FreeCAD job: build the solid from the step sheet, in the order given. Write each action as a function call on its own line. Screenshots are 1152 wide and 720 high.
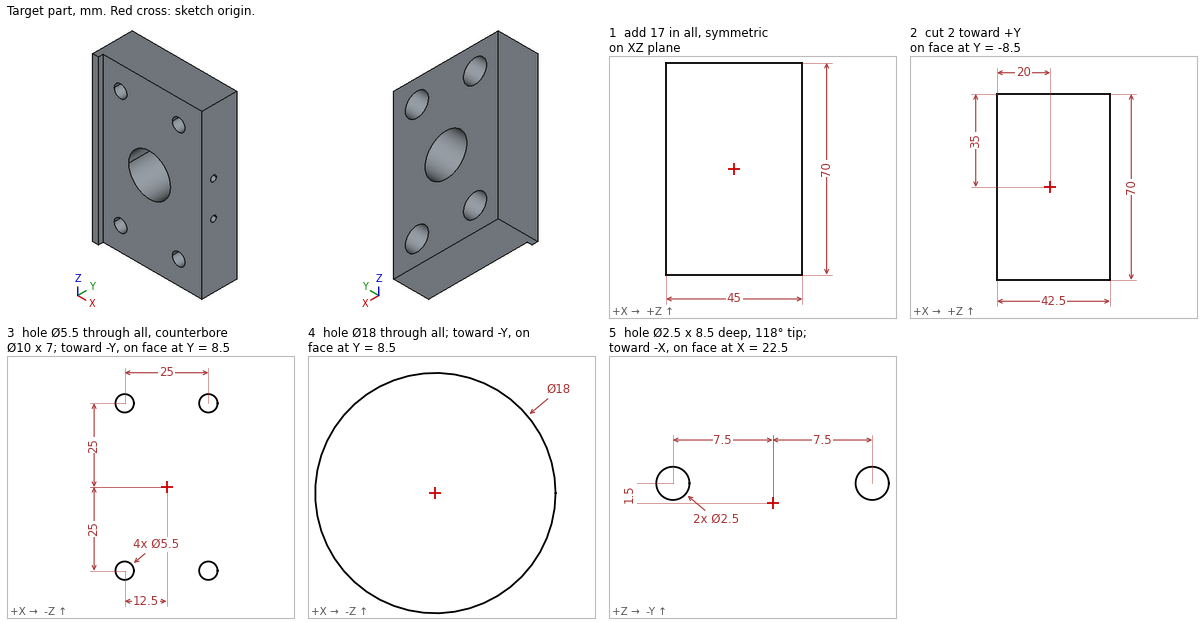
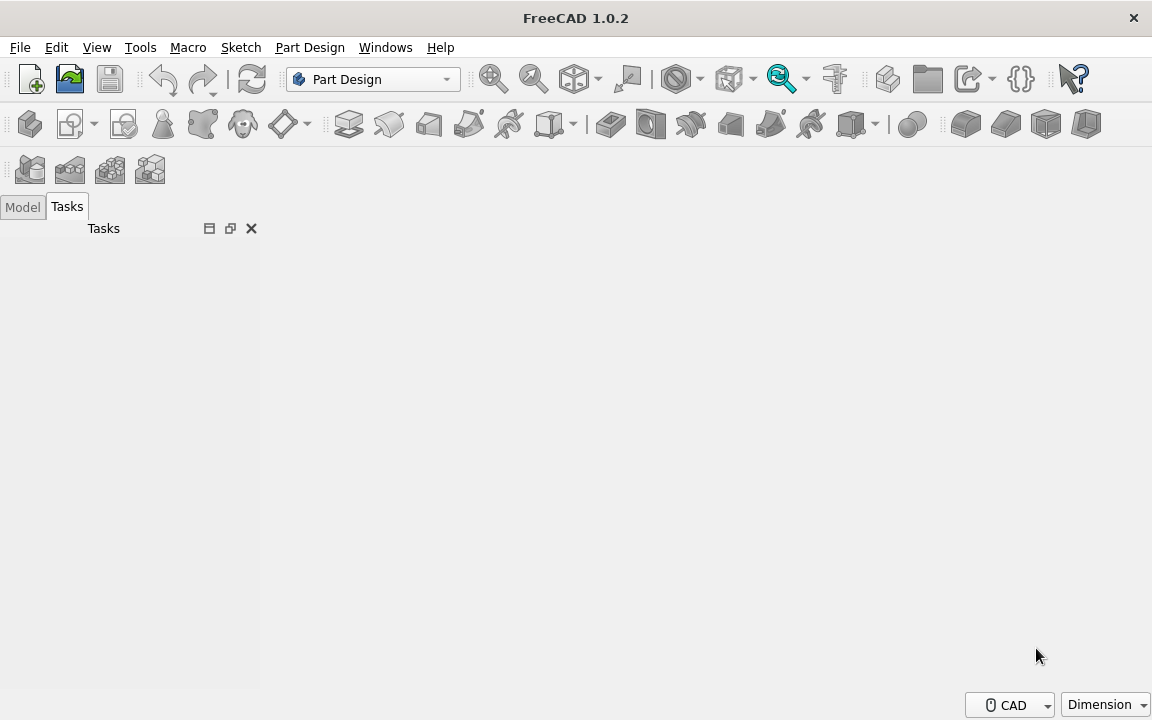
click(30, 80)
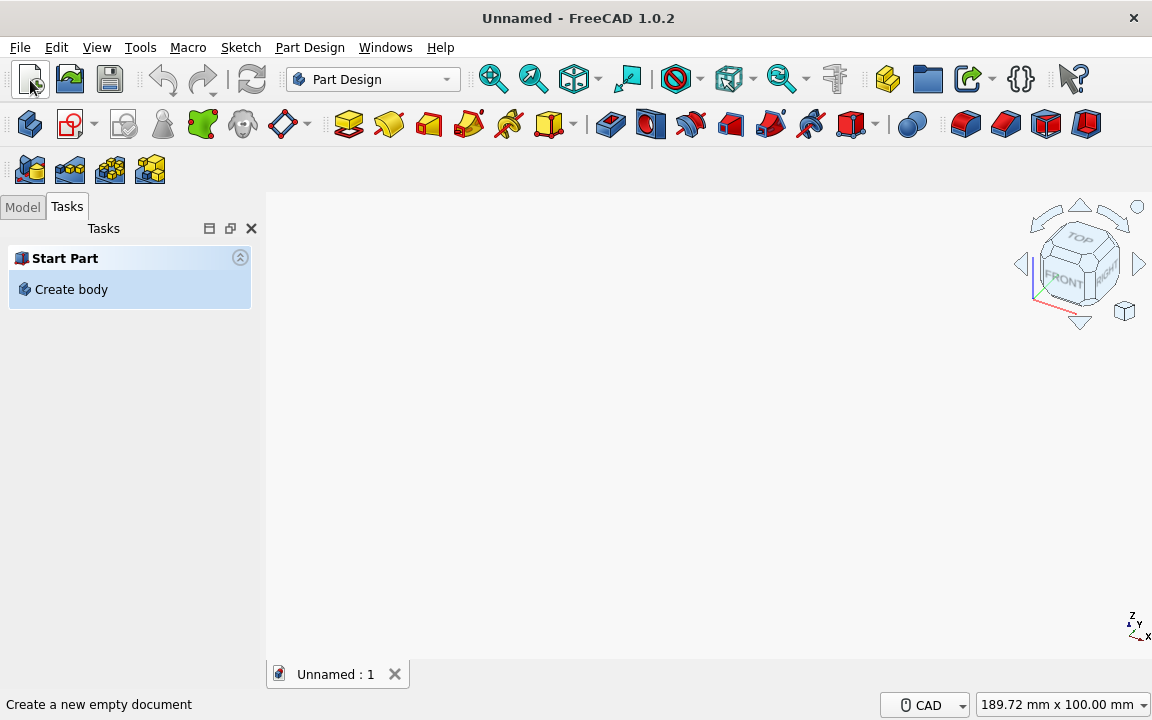
click(70, 124)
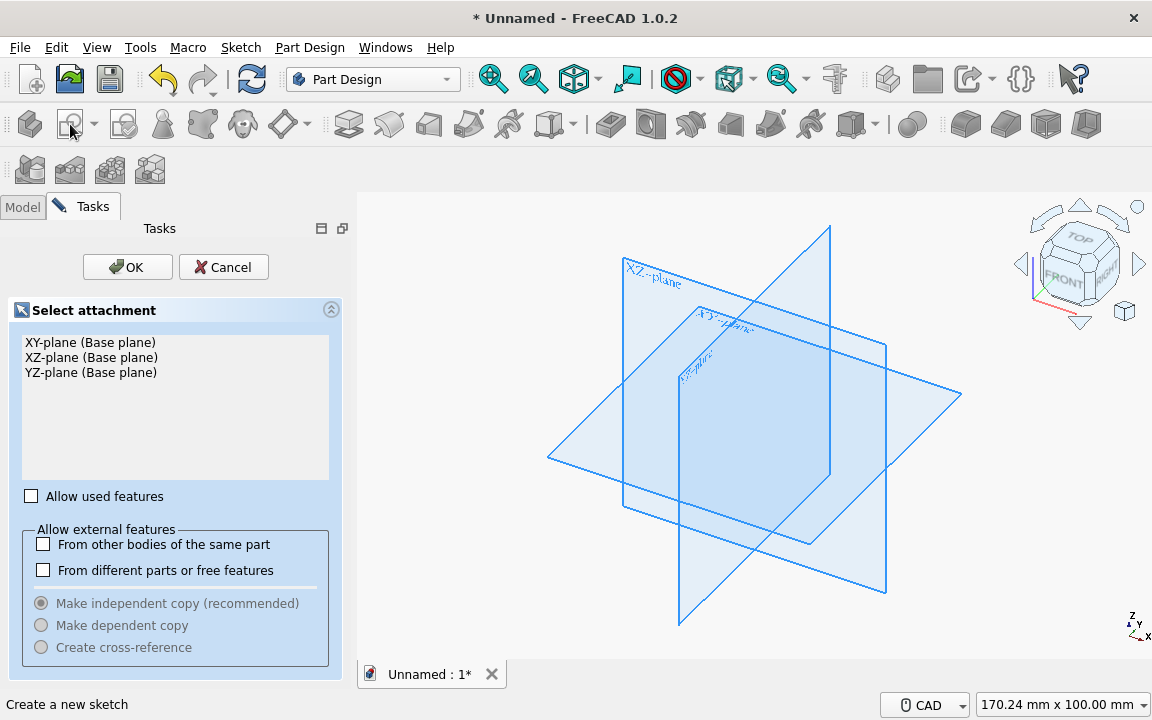
click(82, 358)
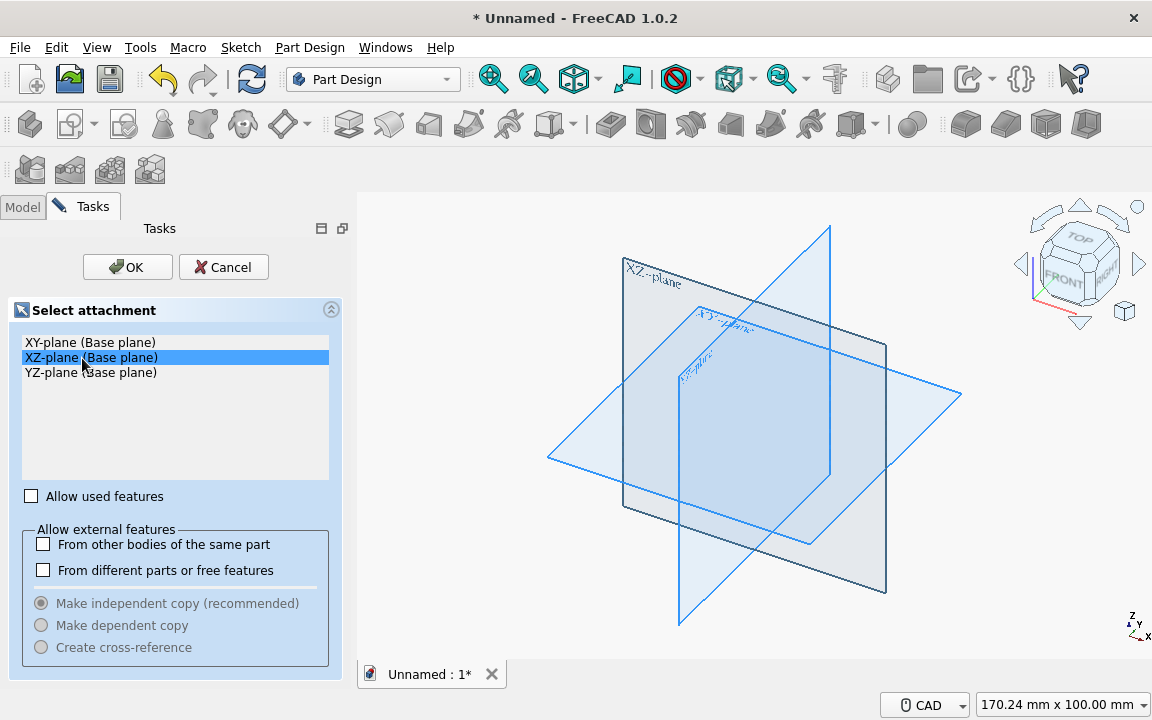
click(128, 267)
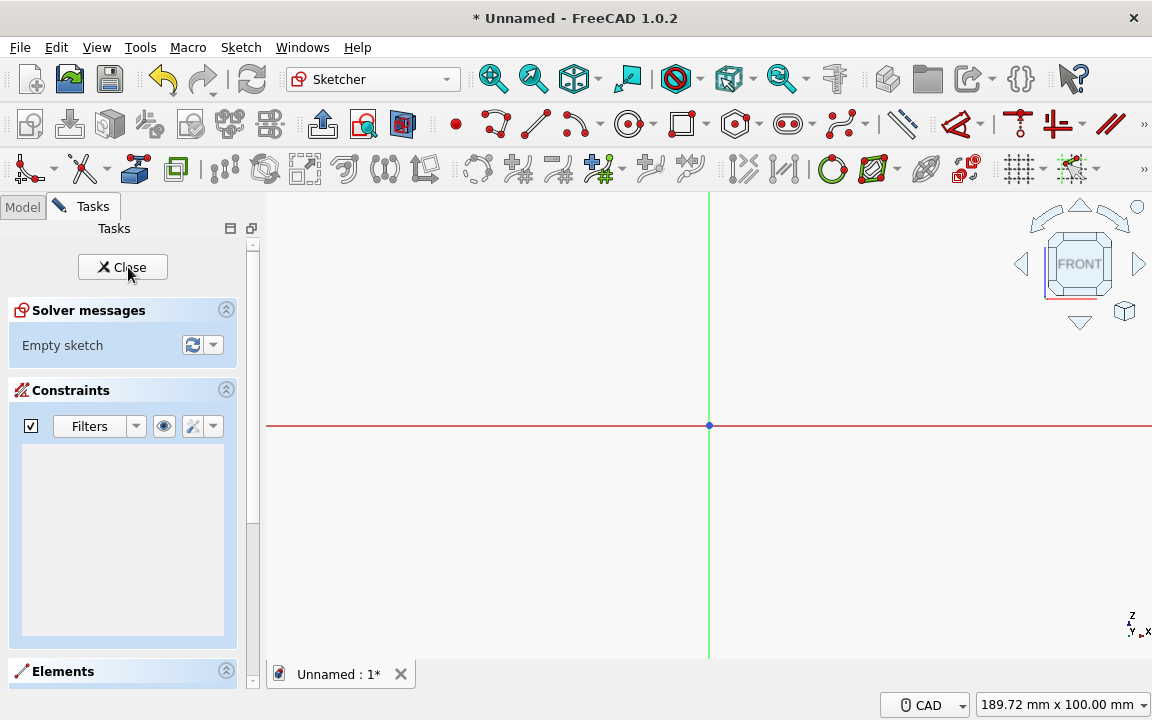
click(708, 124)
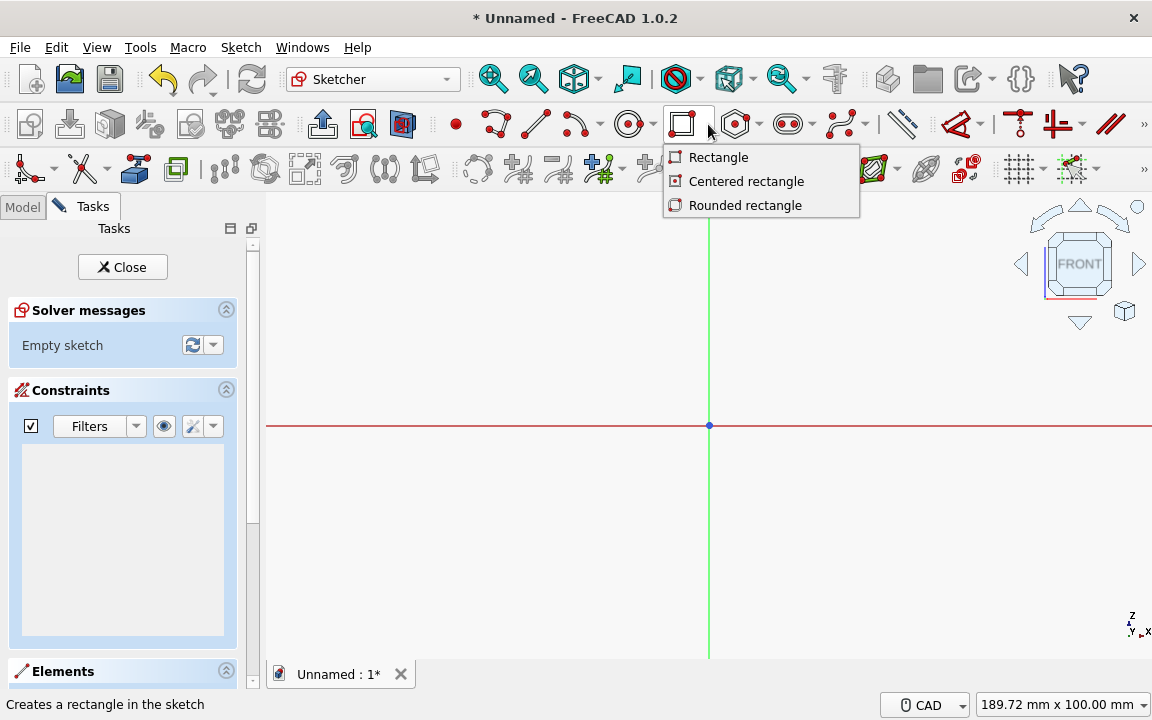
click(762, 181)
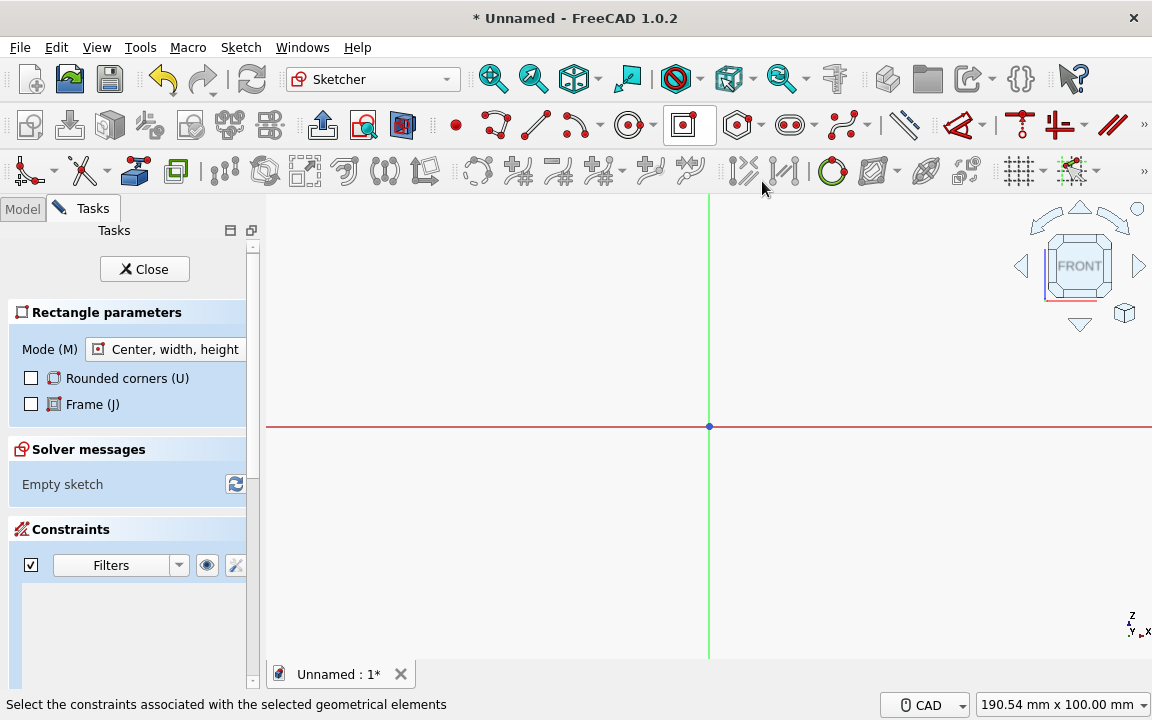
click(709, 426)
move(814, 264)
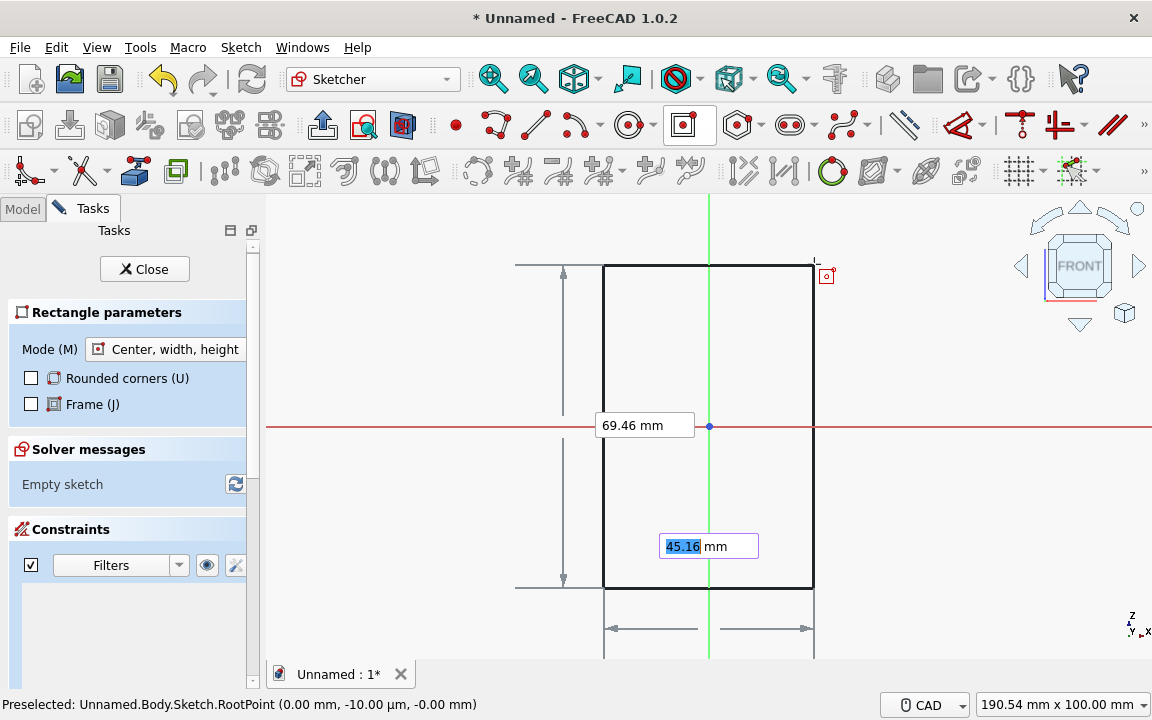
text(45)
key(Tab)
text(70)
key(Return)
key(Escape)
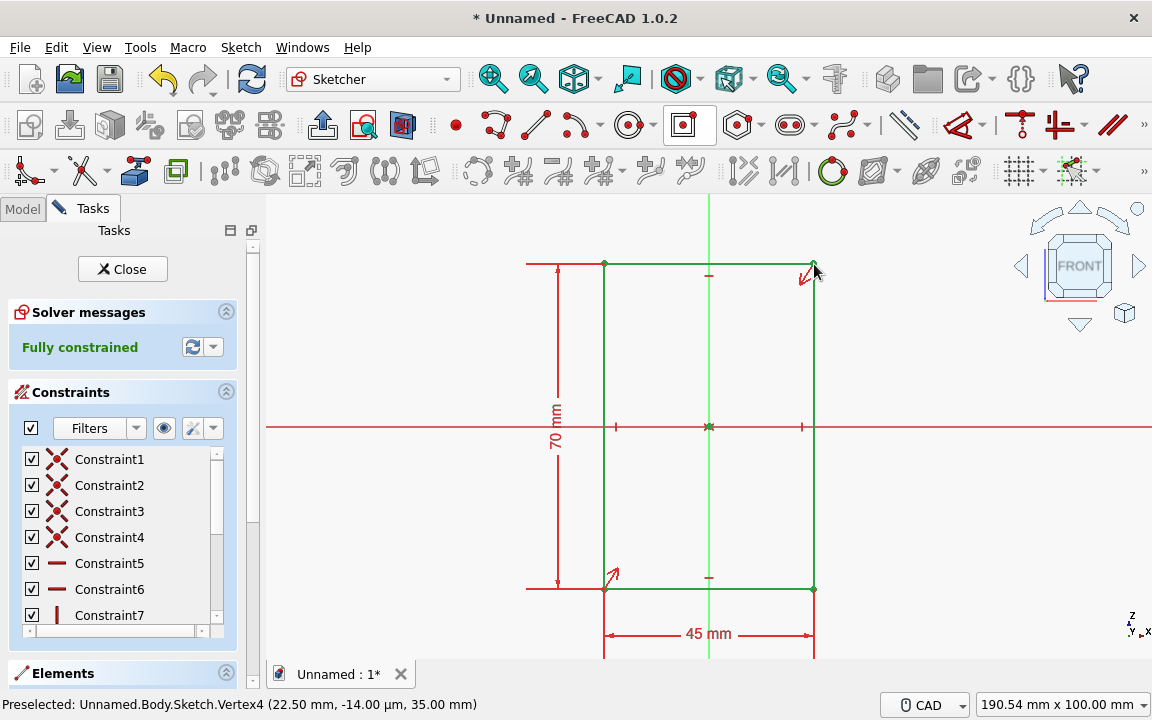
click(123, 269)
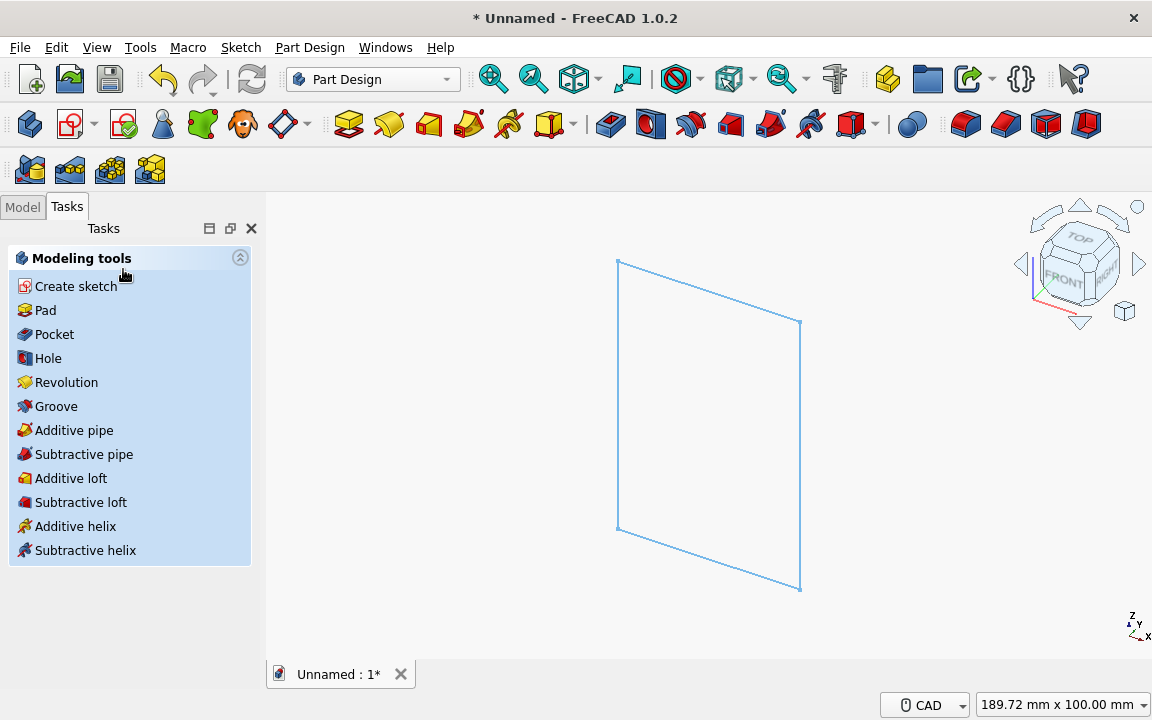
click(350, 124)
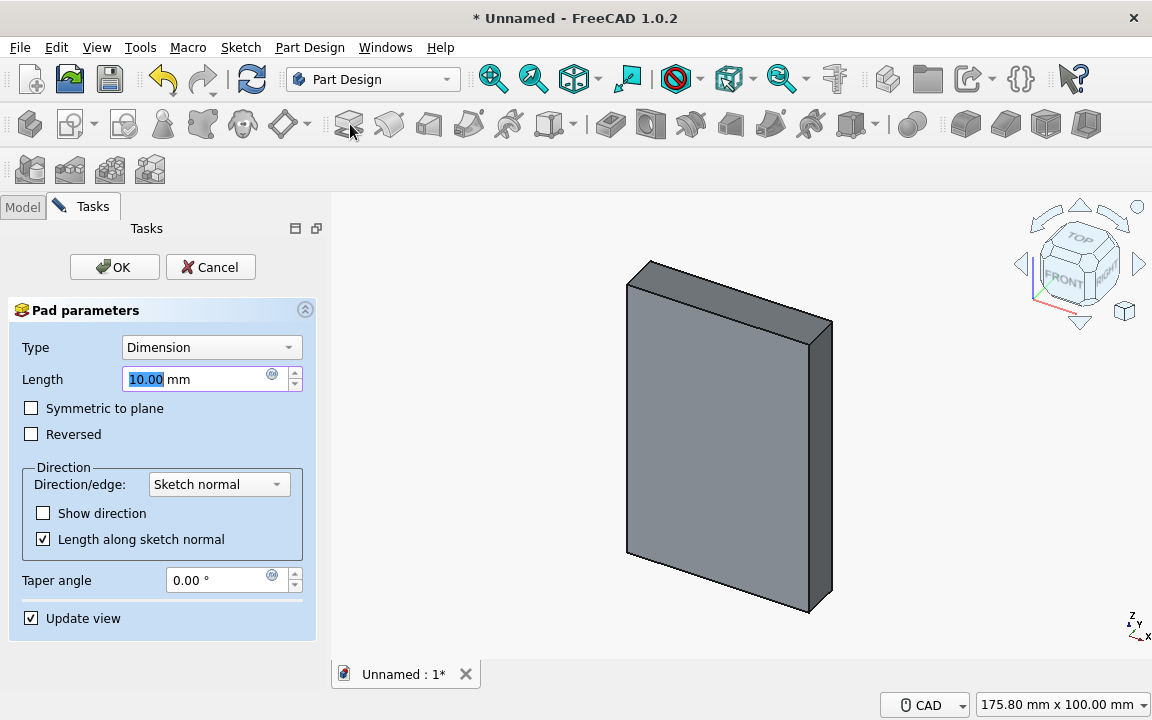
text(17)
key(Tab)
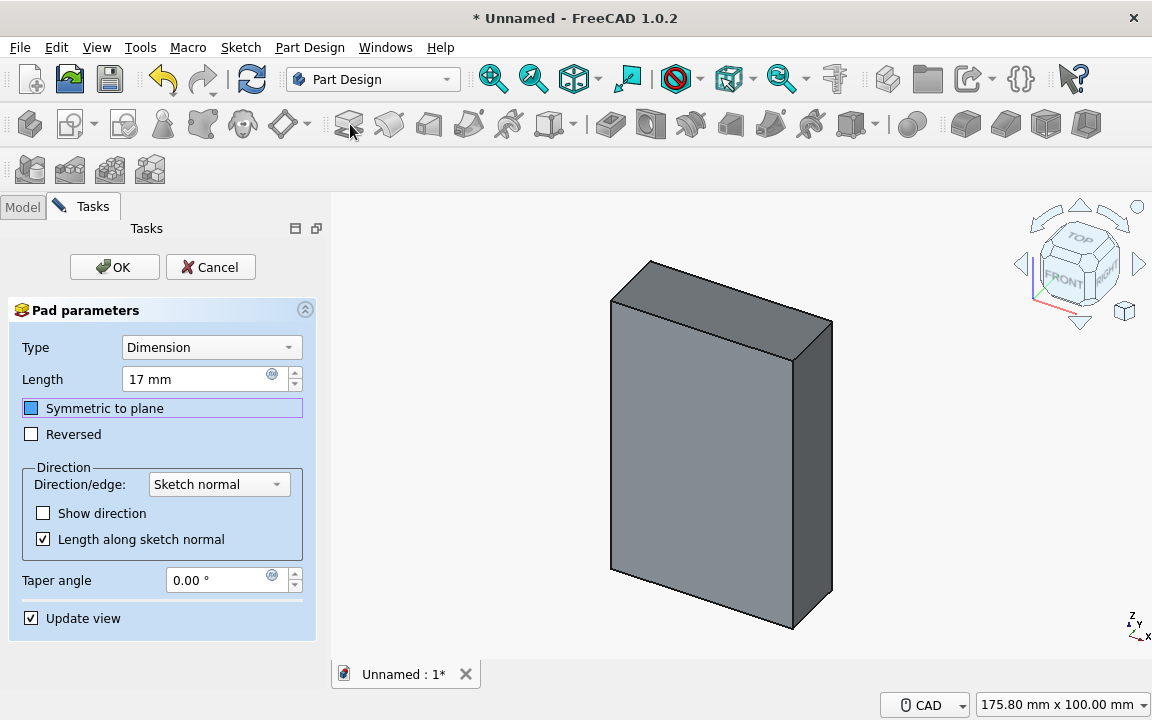
click(30, 408)